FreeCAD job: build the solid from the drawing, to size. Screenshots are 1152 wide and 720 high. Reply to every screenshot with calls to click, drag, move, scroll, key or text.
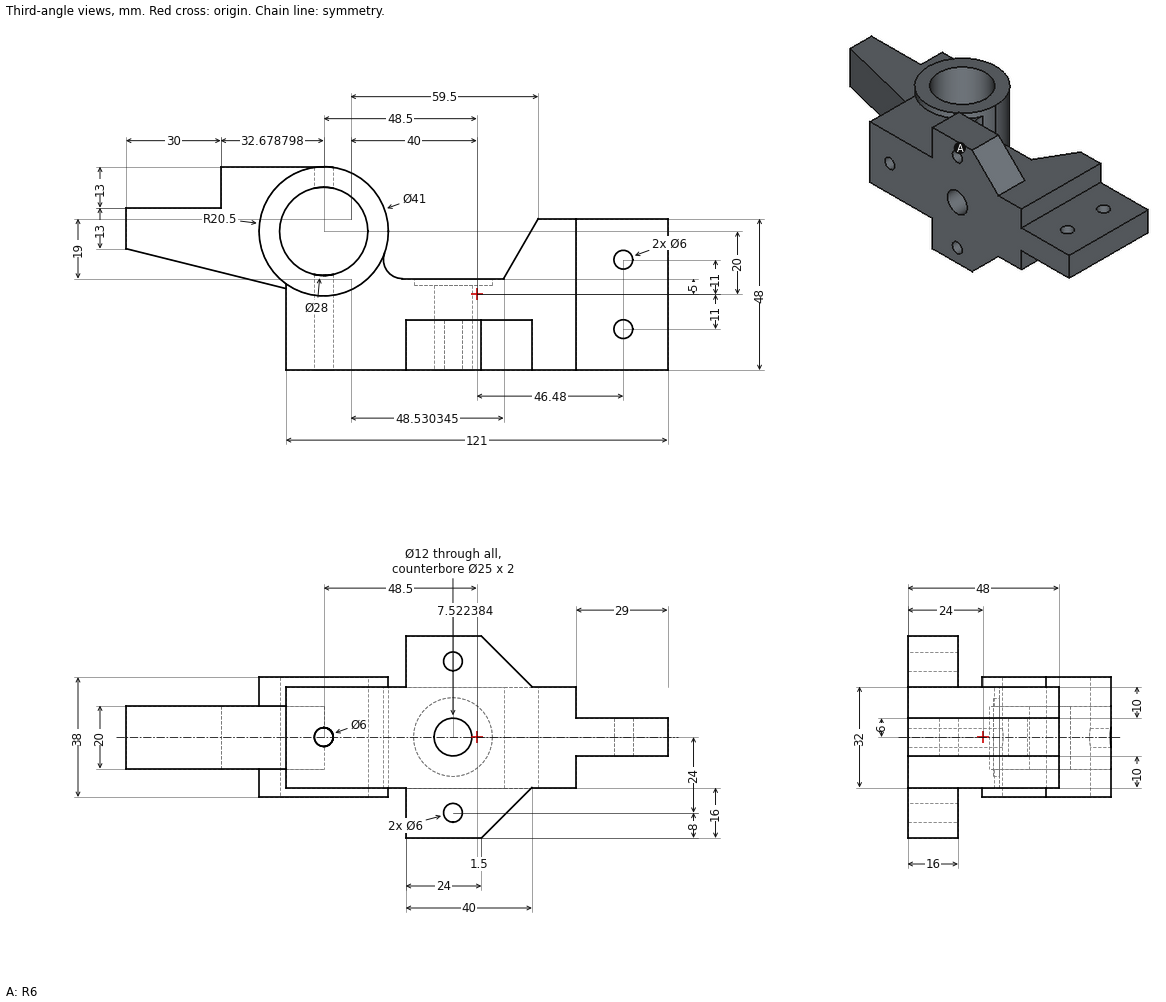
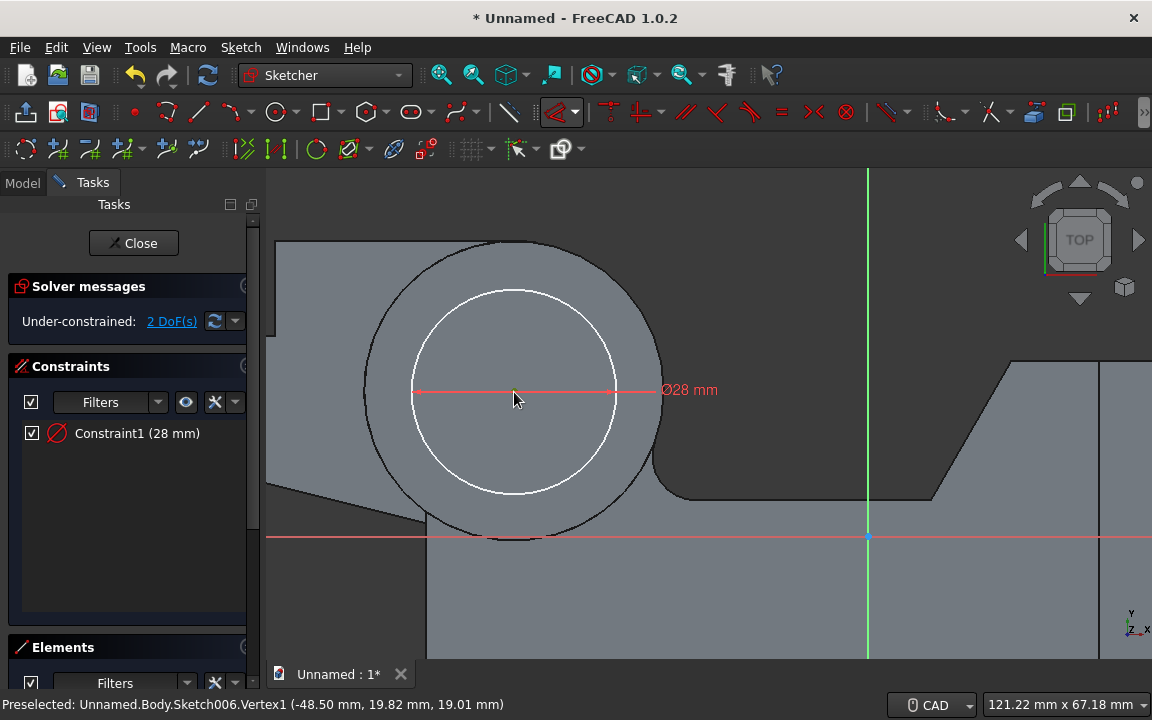
key(i)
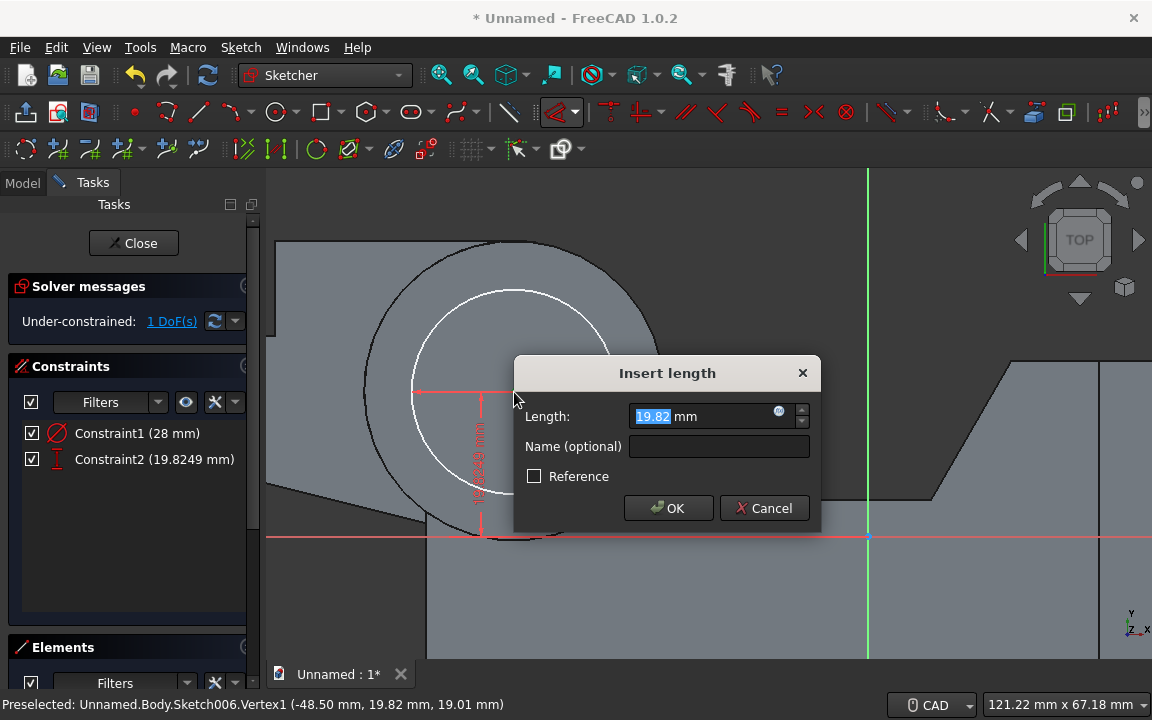
text(20)
key(Return)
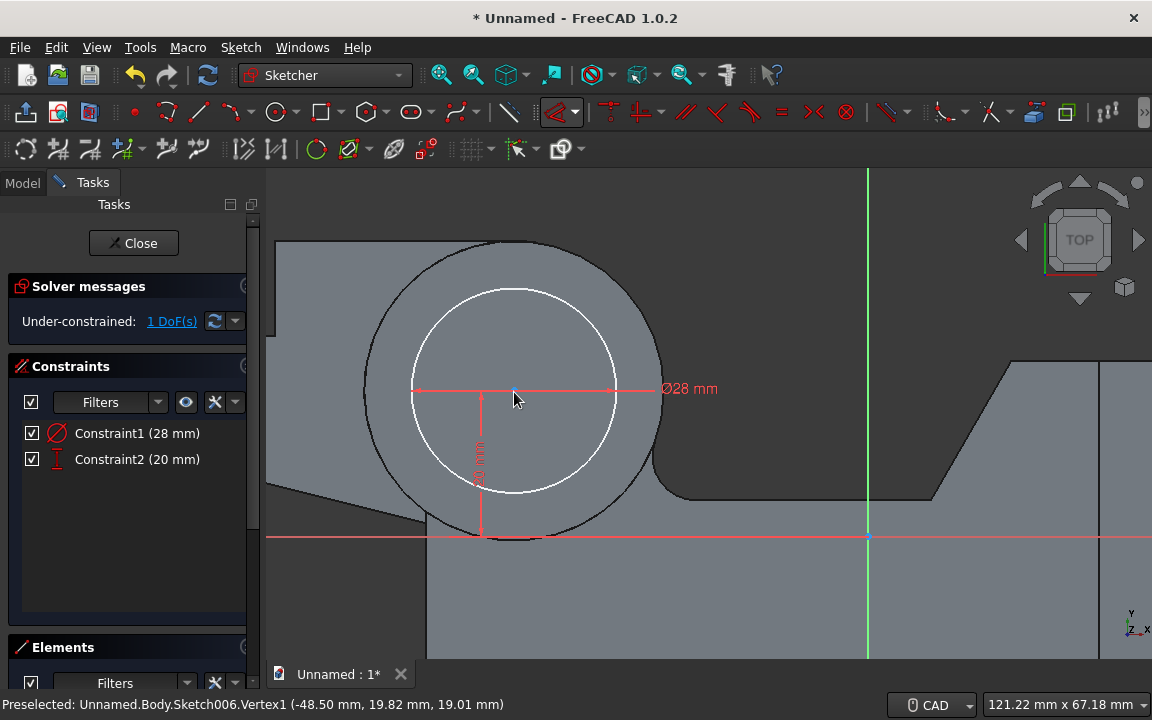
click(514, 391)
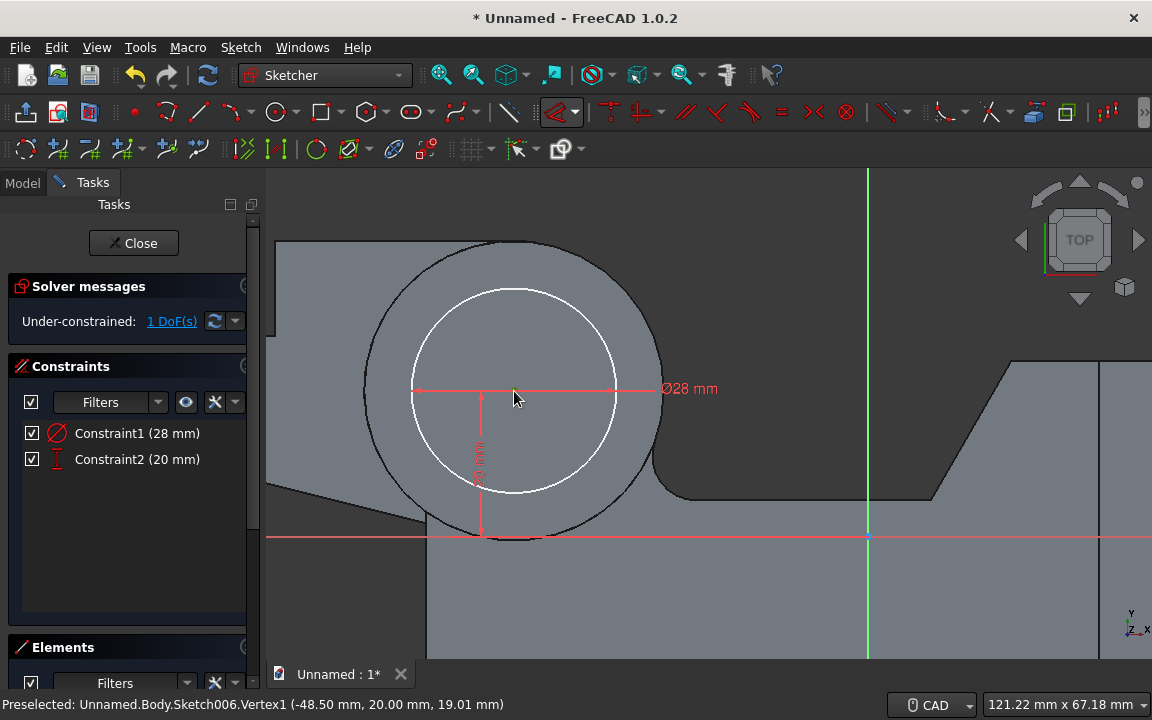
key(l)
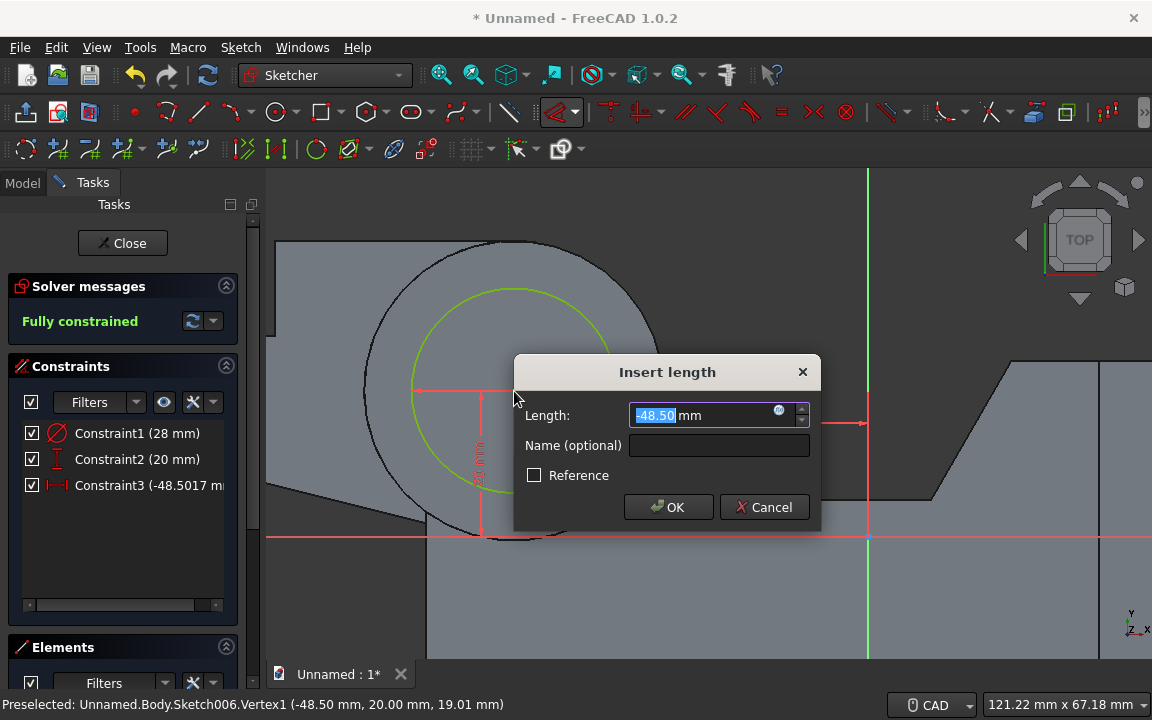
text(-48.5)
key(Return)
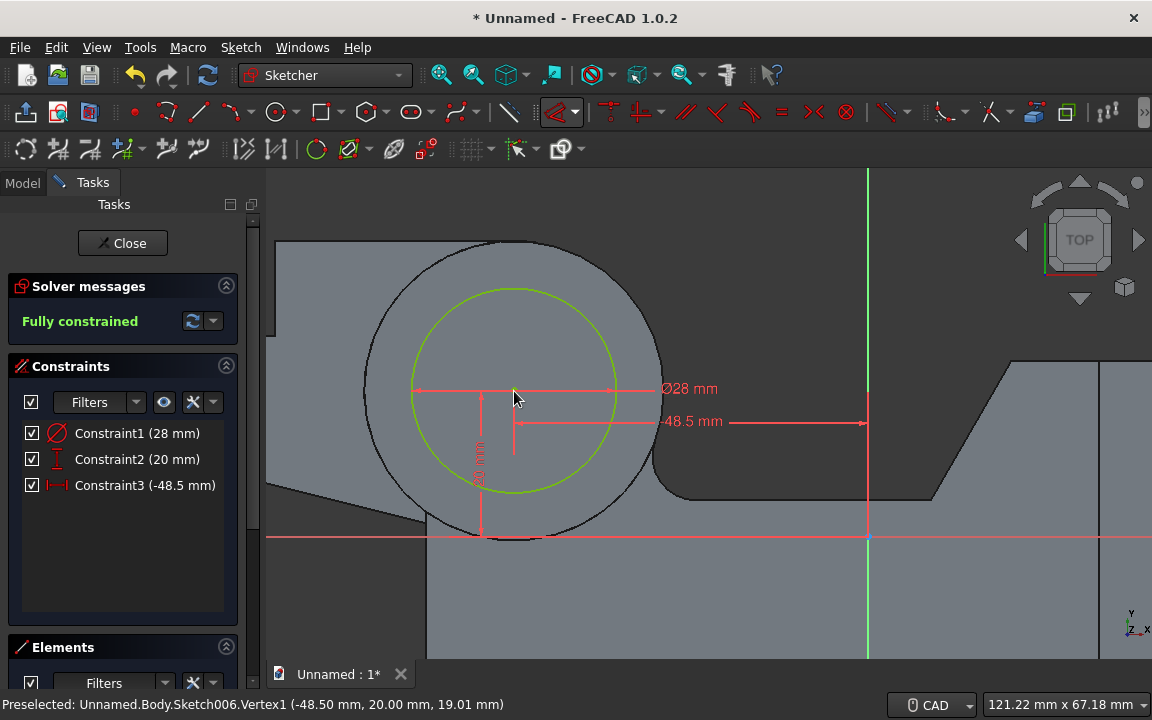
click(123, 243)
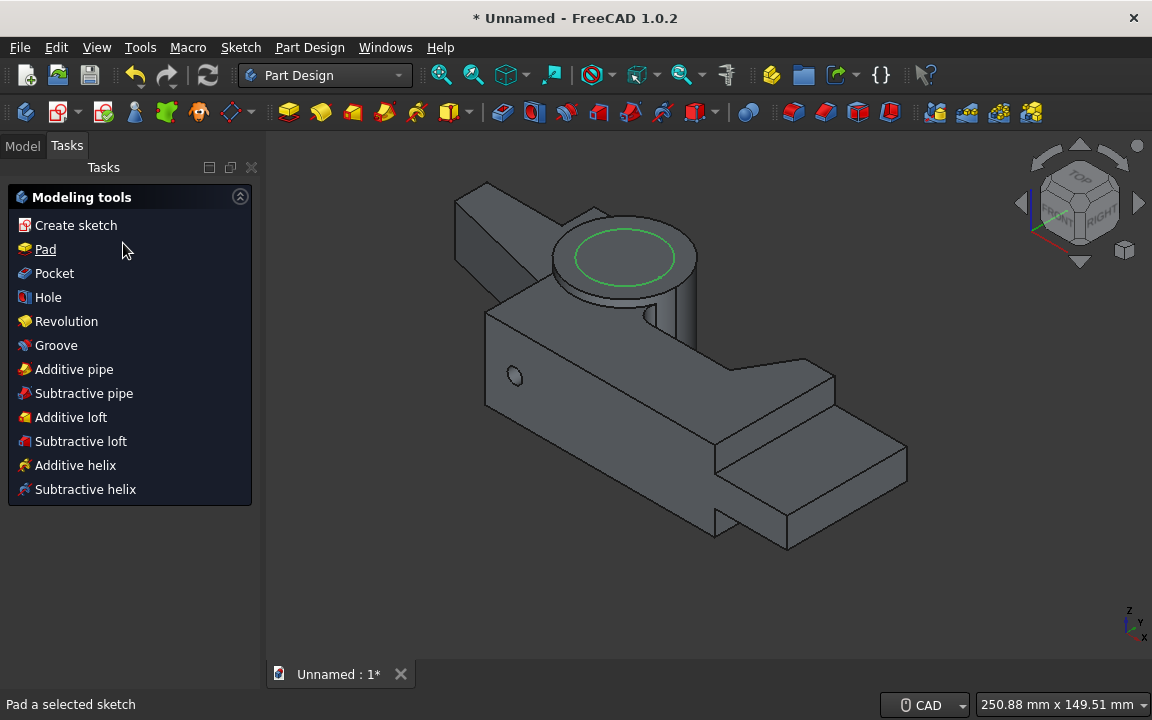
click(504, 112)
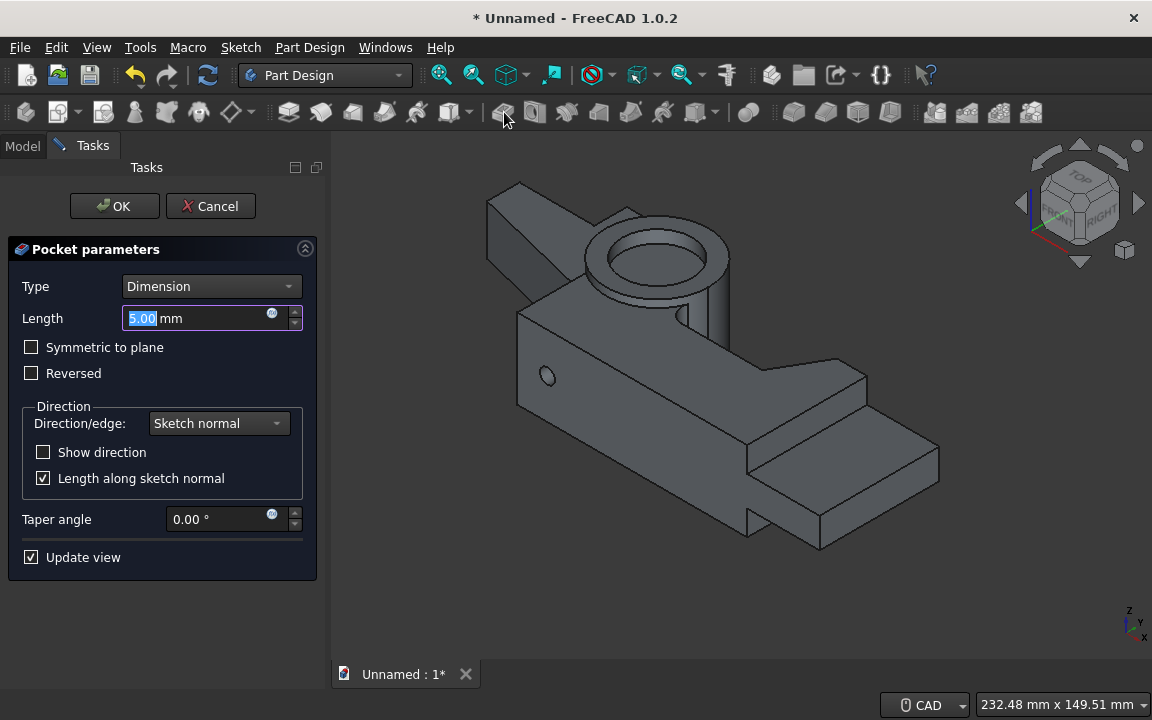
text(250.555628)
key(Tab)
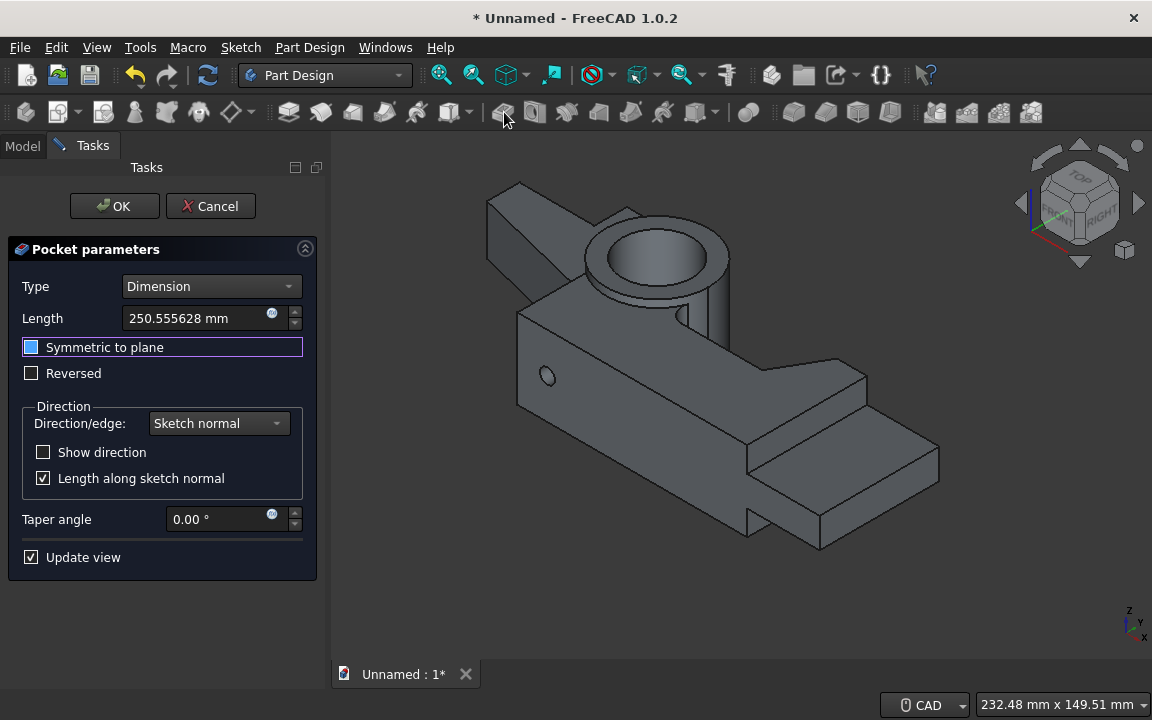
click(30, 347)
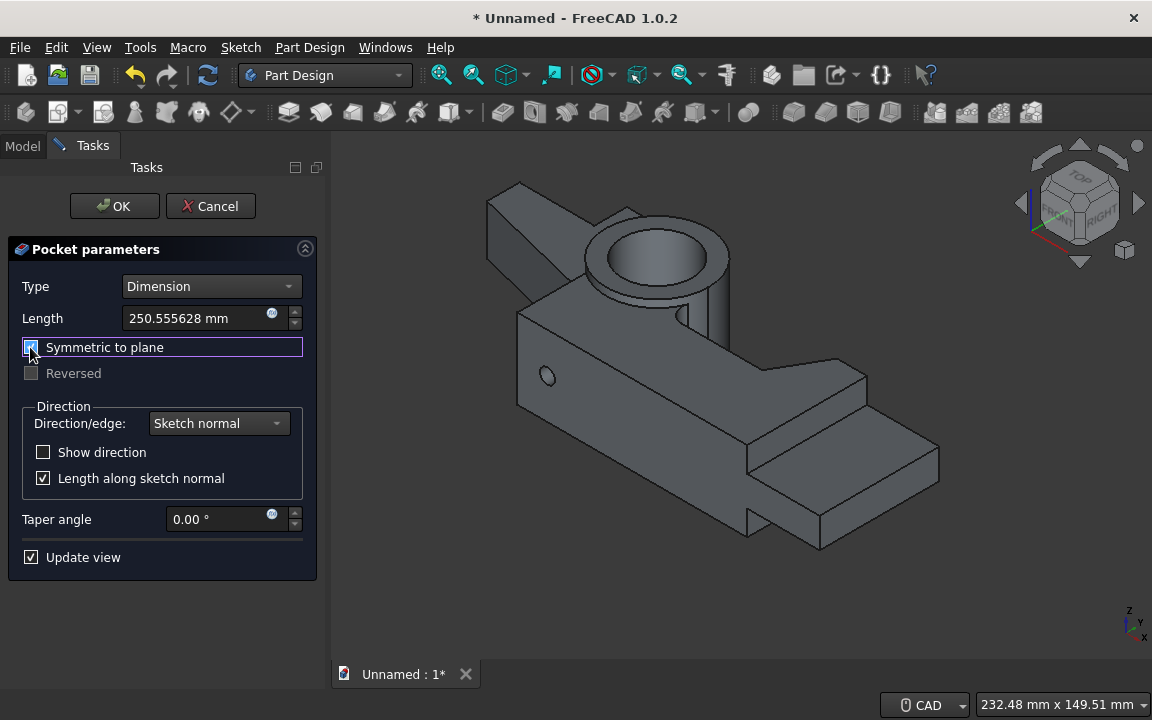
click(115, 206)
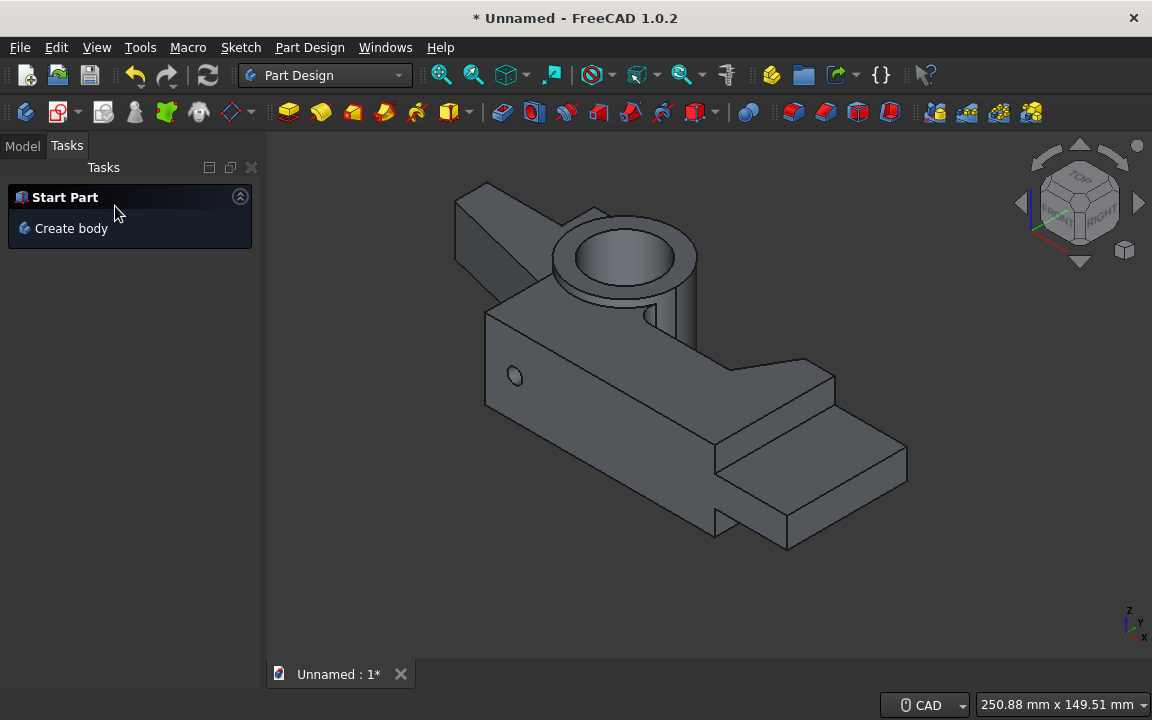
key(4)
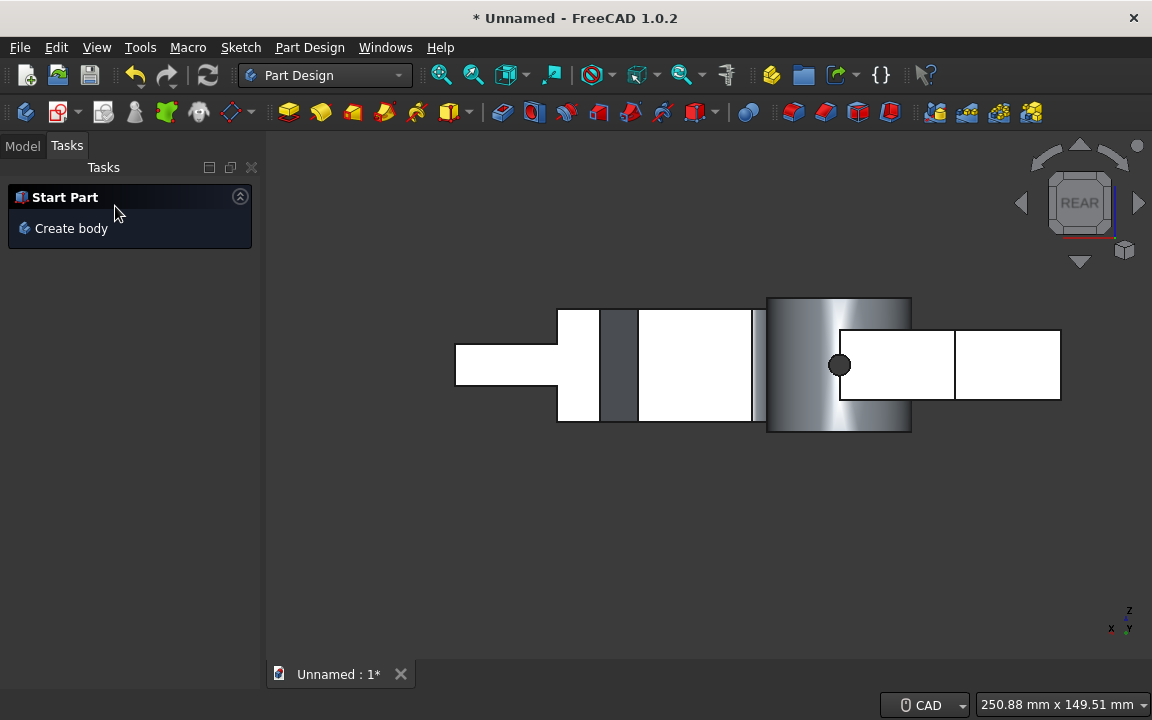
click(695, 364)